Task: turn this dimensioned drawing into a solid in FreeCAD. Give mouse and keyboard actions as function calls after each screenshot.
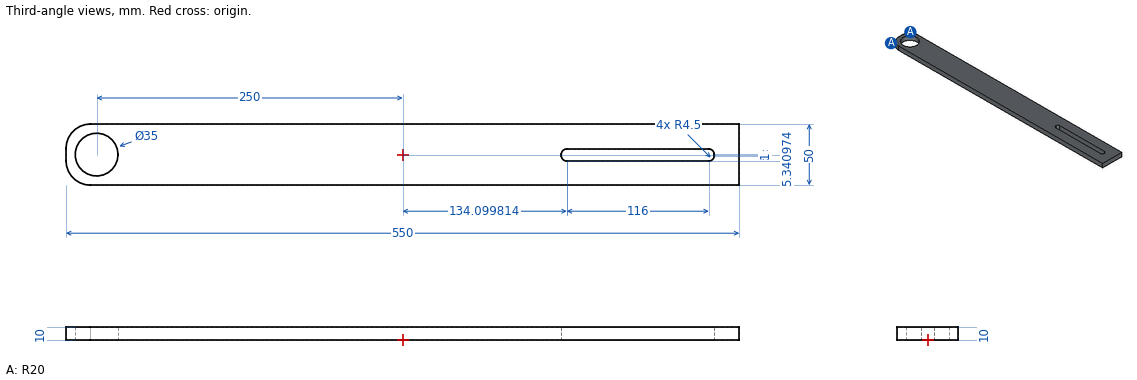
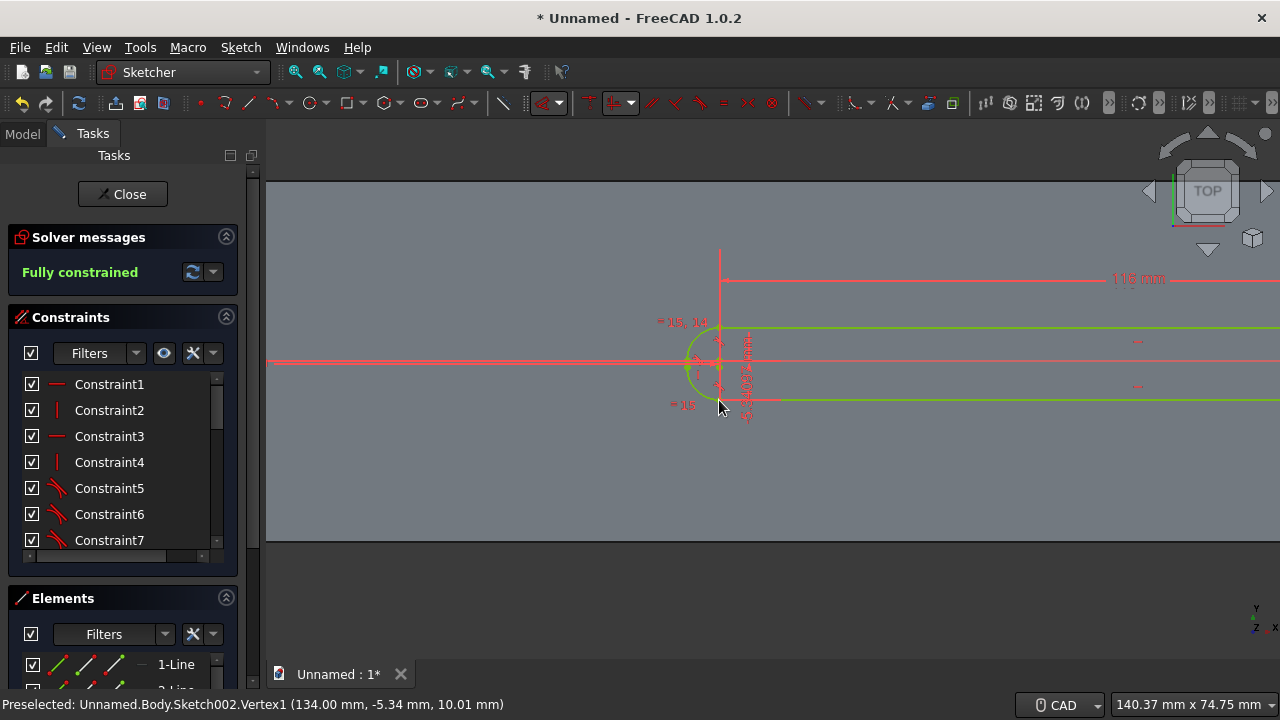
click(123, 194)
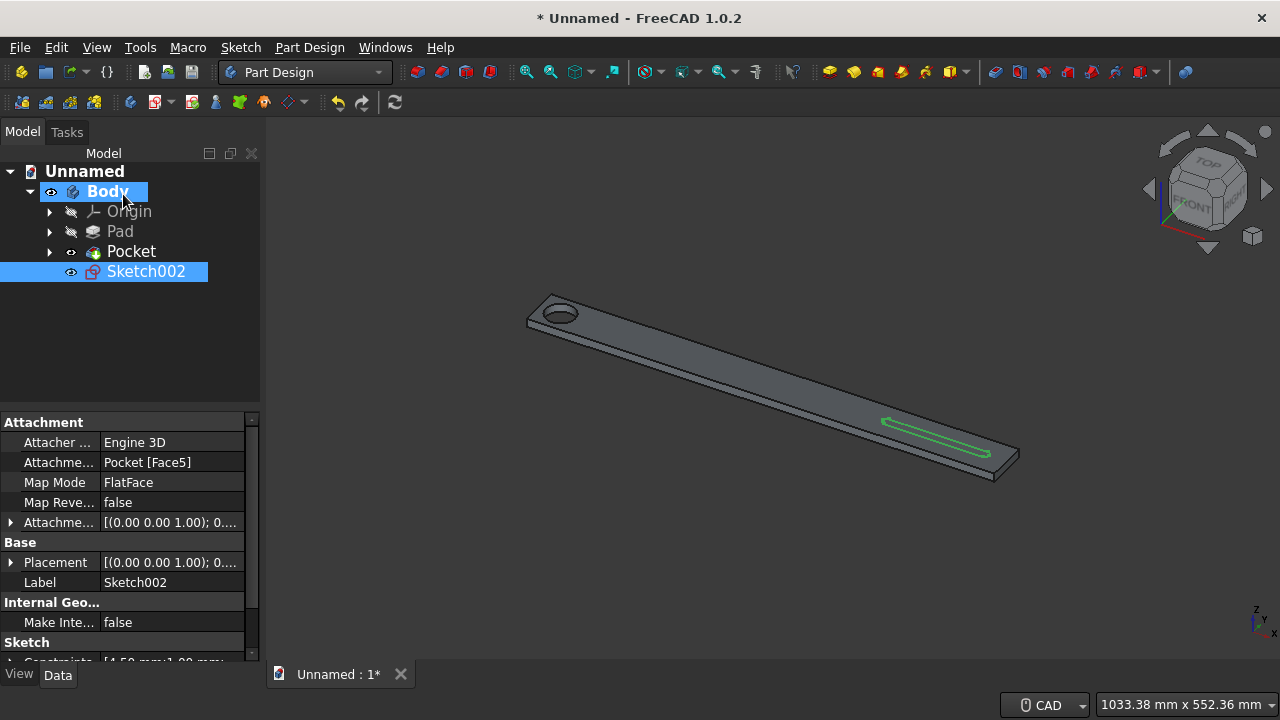
click(996, 72)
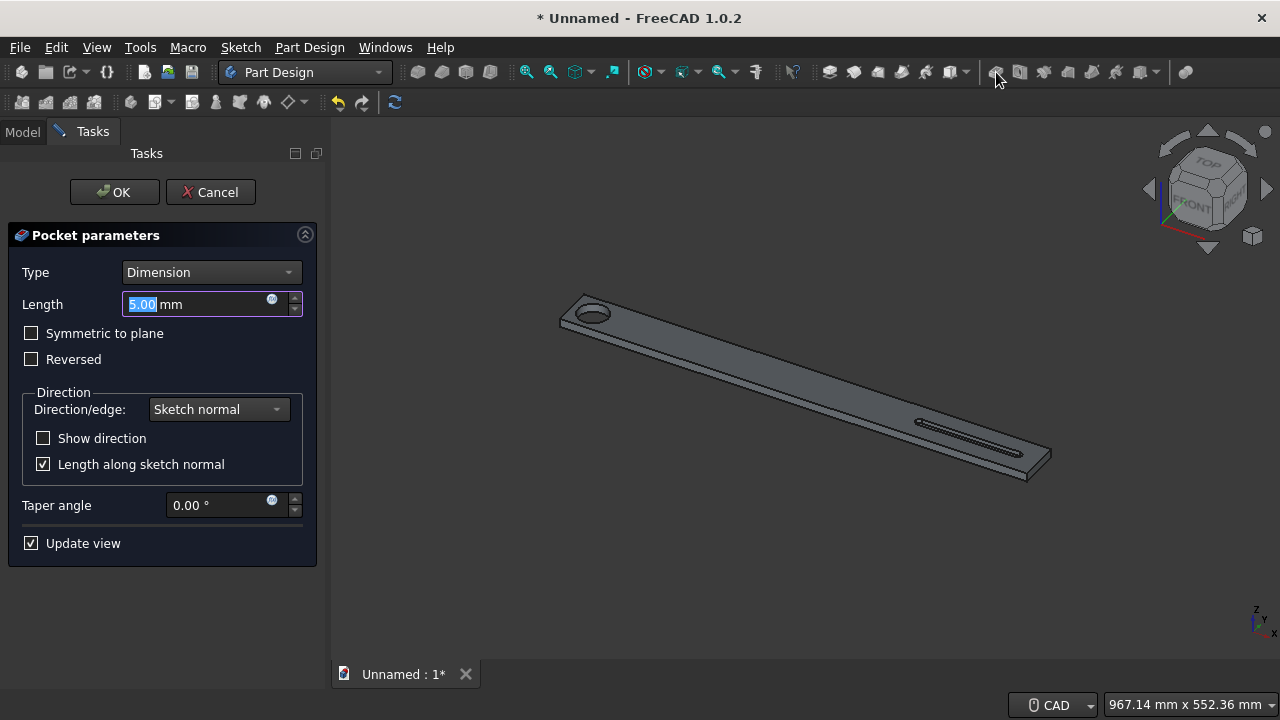
text(10)
key(Tab)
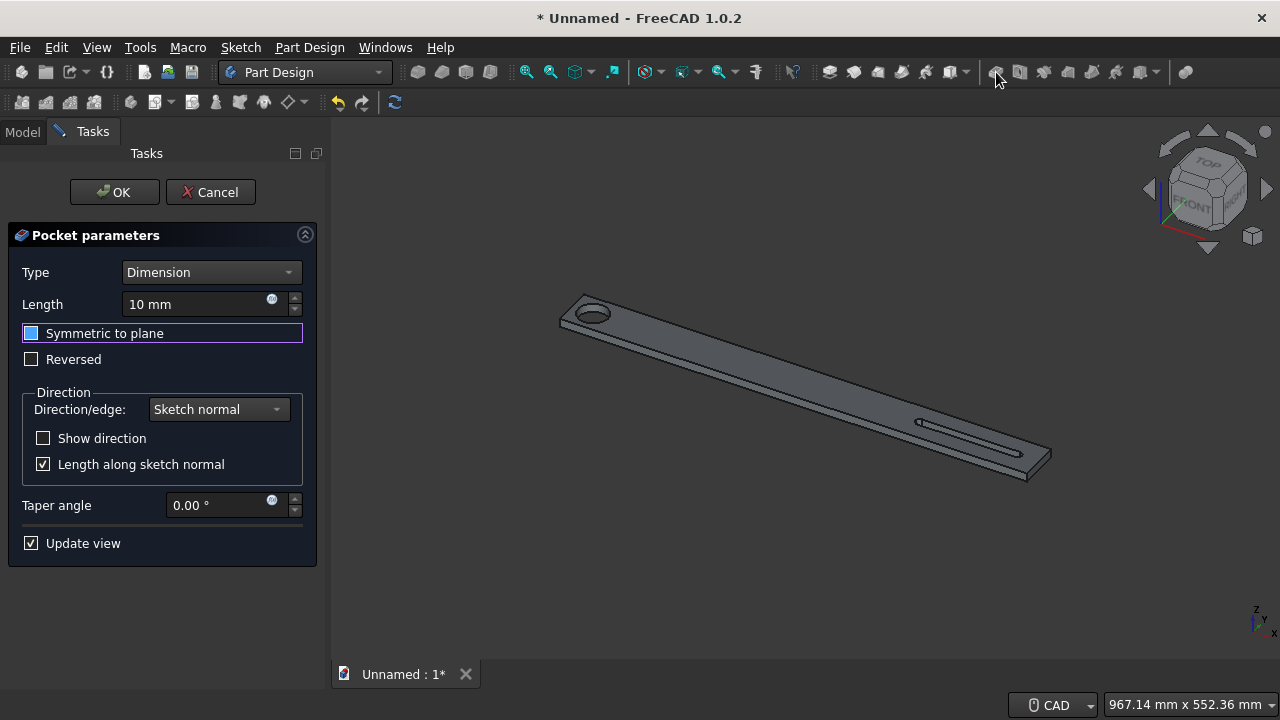
click(115, 192)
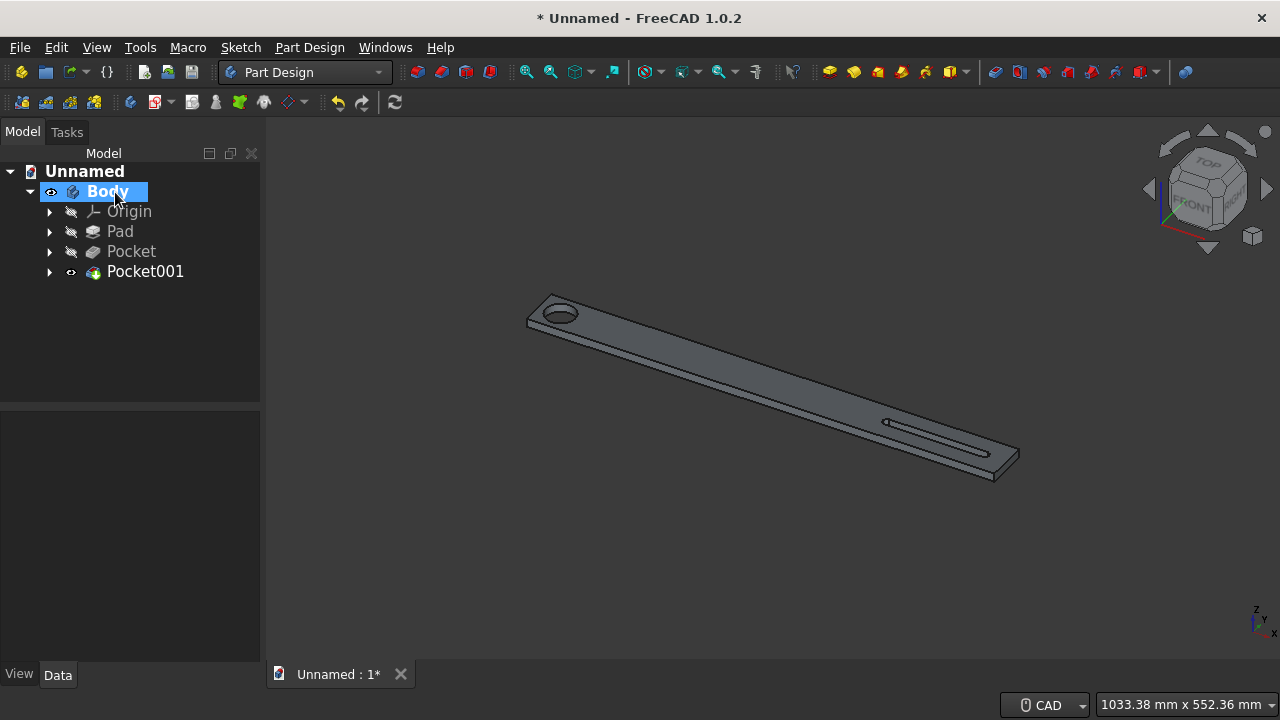
scroll(552, 297, up, 8)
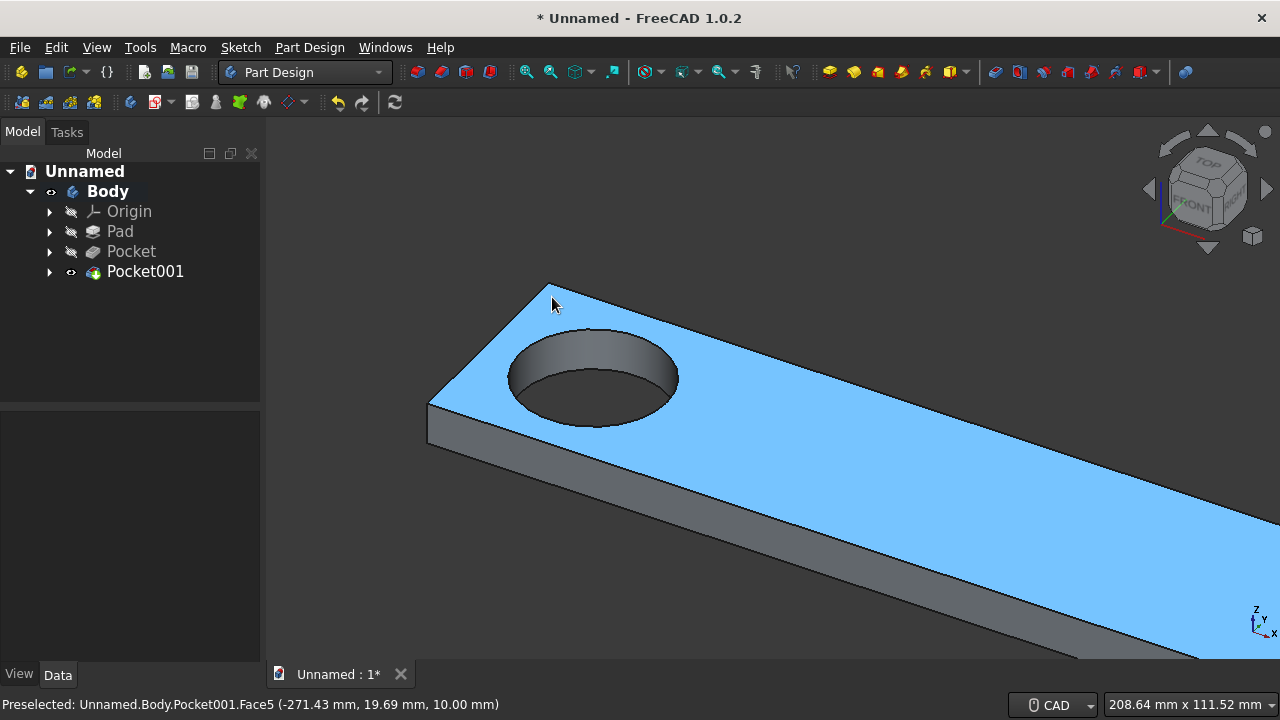
click(528, 72)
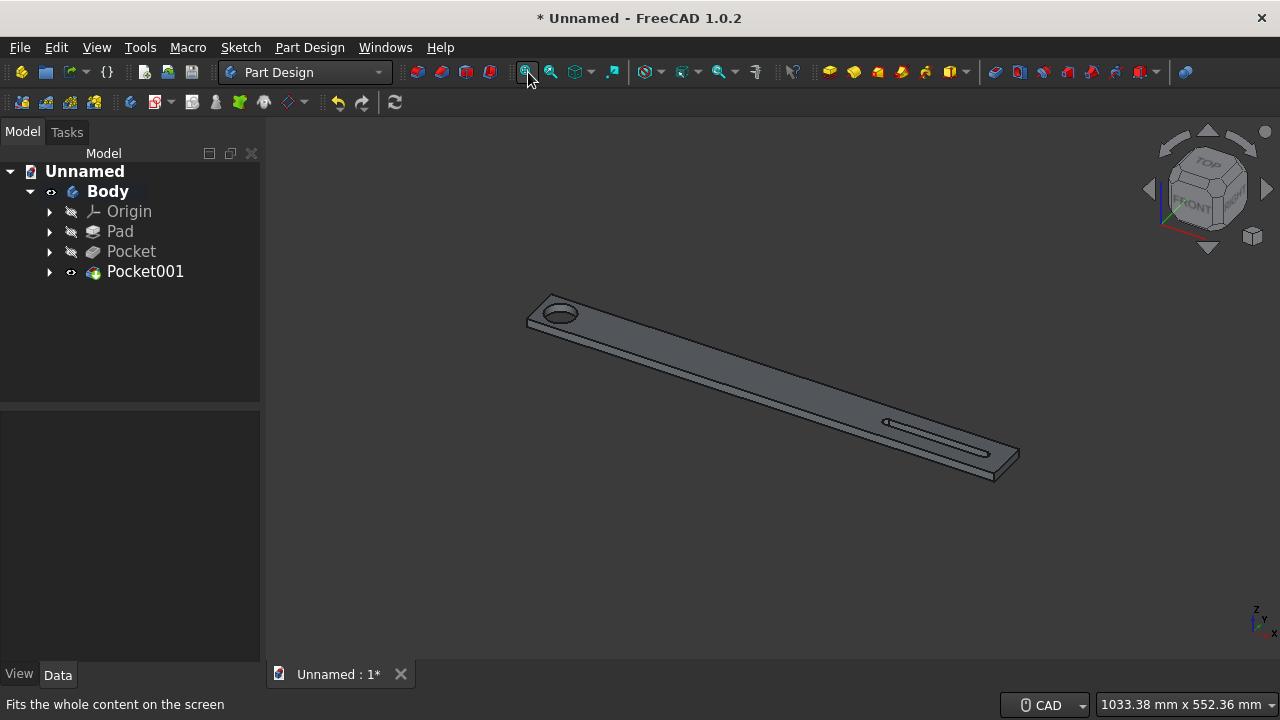
key(0)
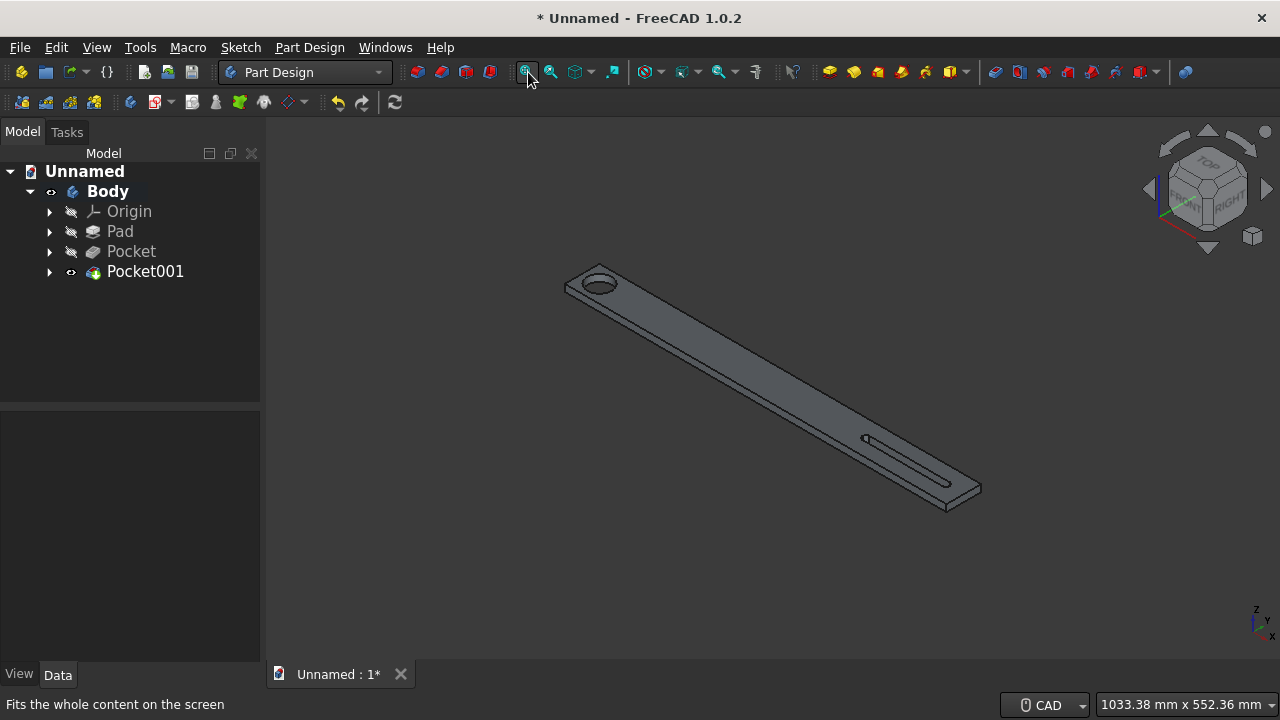
scroll(600, 267, up, 8)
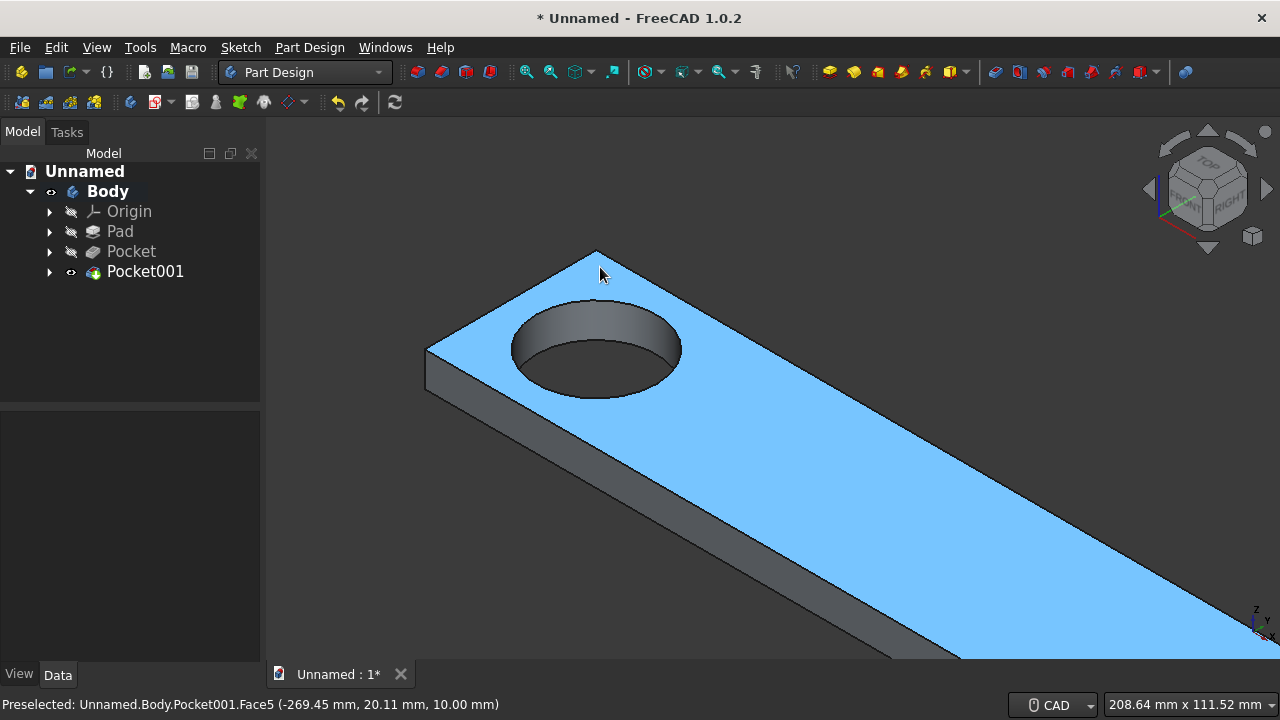
click(528, 72)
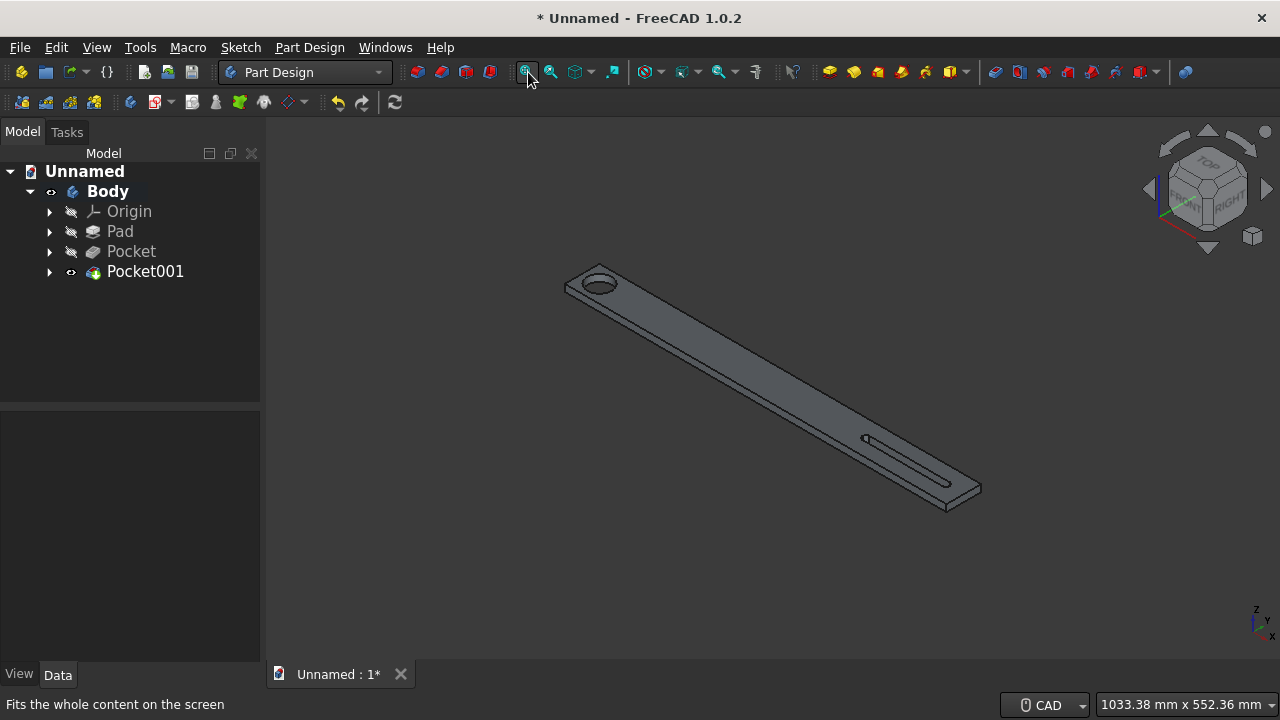
key(2)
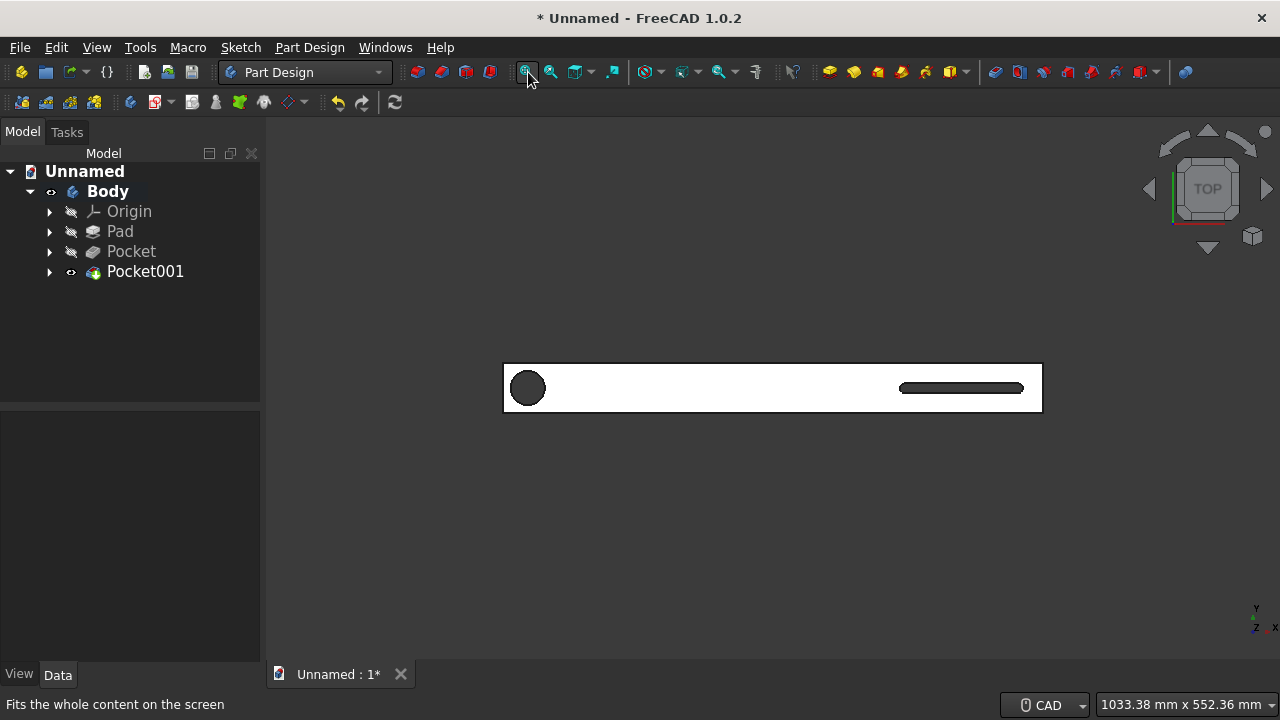
scroll(503, 362, up, 8)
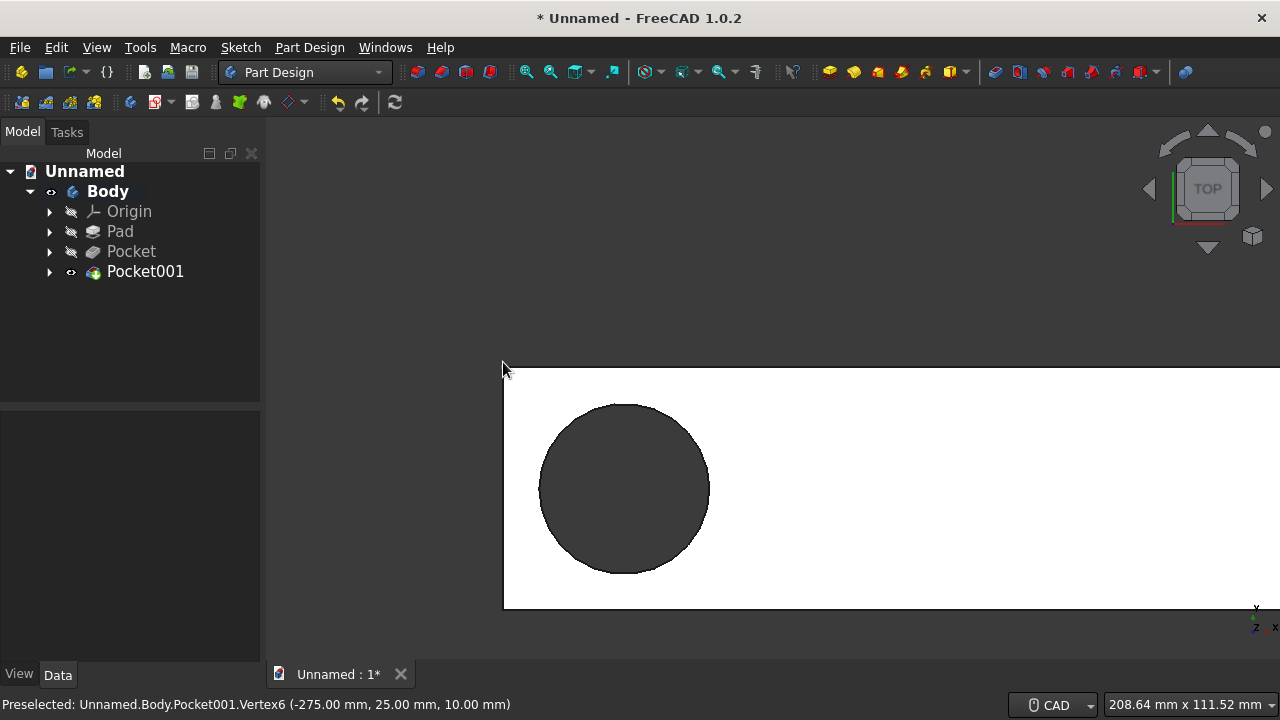
click(528, 72)